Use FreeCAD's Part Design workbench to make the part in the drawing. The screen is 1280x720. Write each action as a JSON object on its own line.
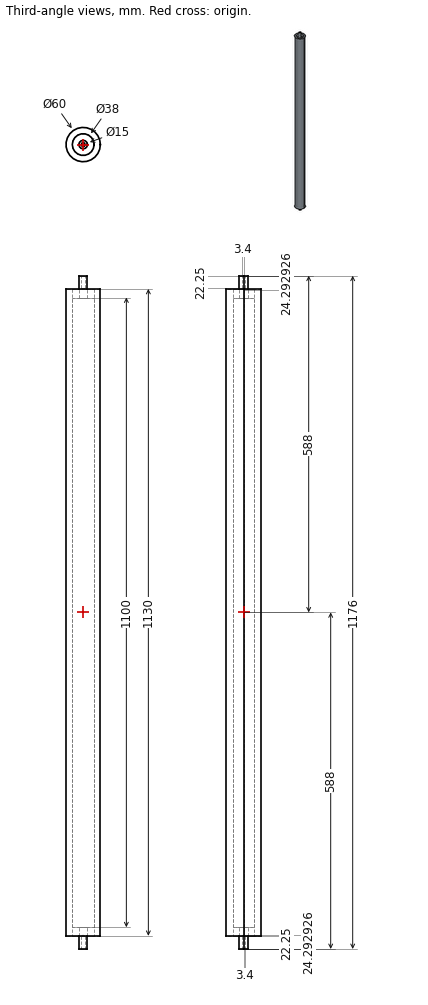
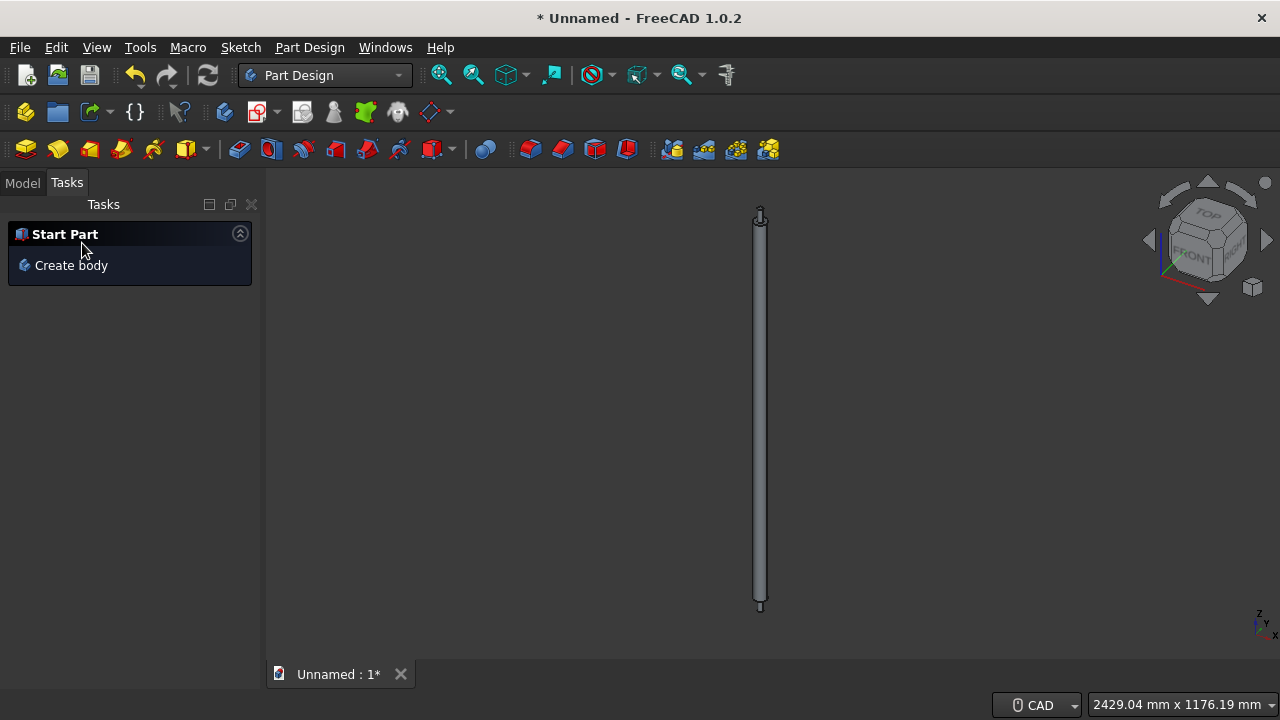
{"action": "left_click", "coordinate": [258, 112]}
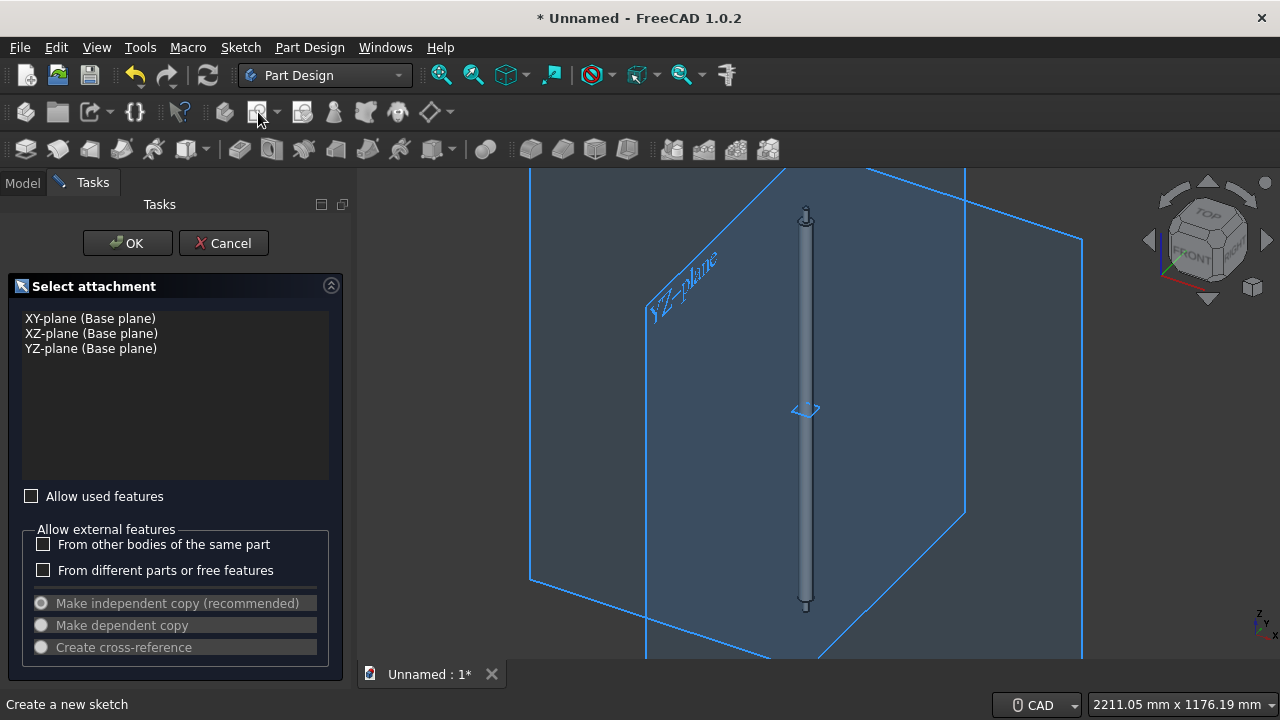
{"action": "left_click", "coordinate": [82, 348]}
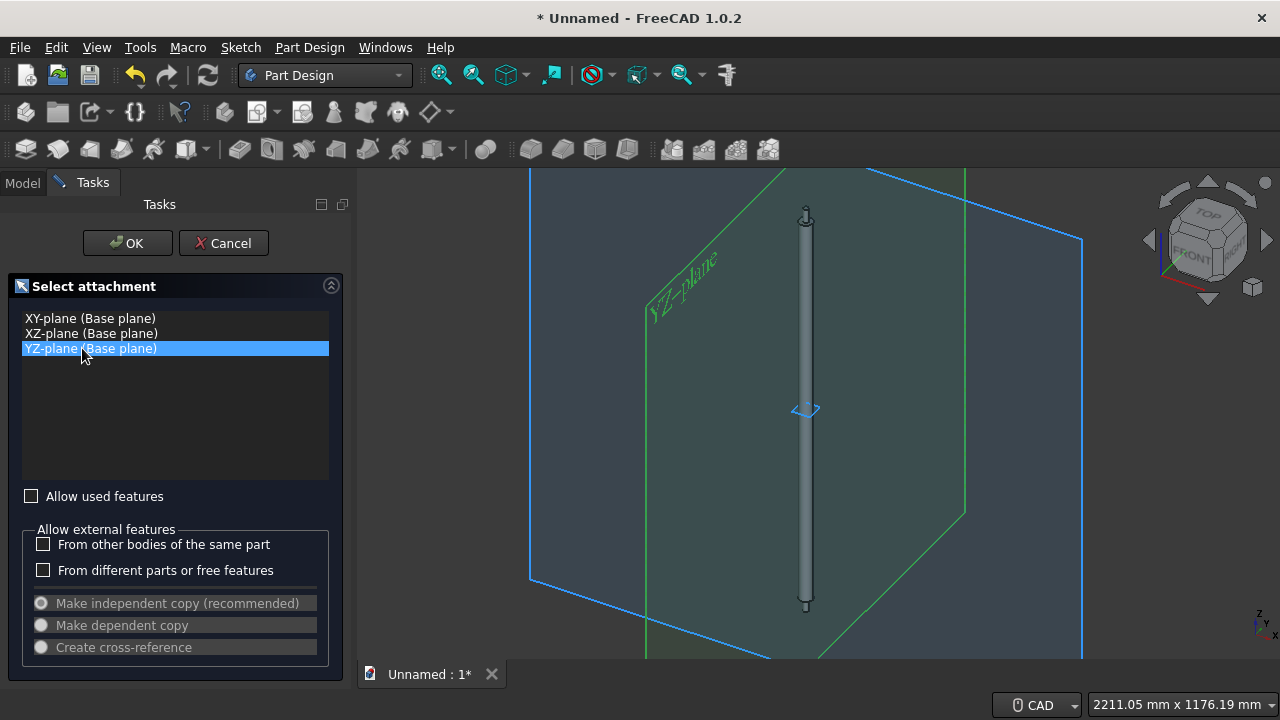
{"action": "left_click", "coordinate": [128, 243]}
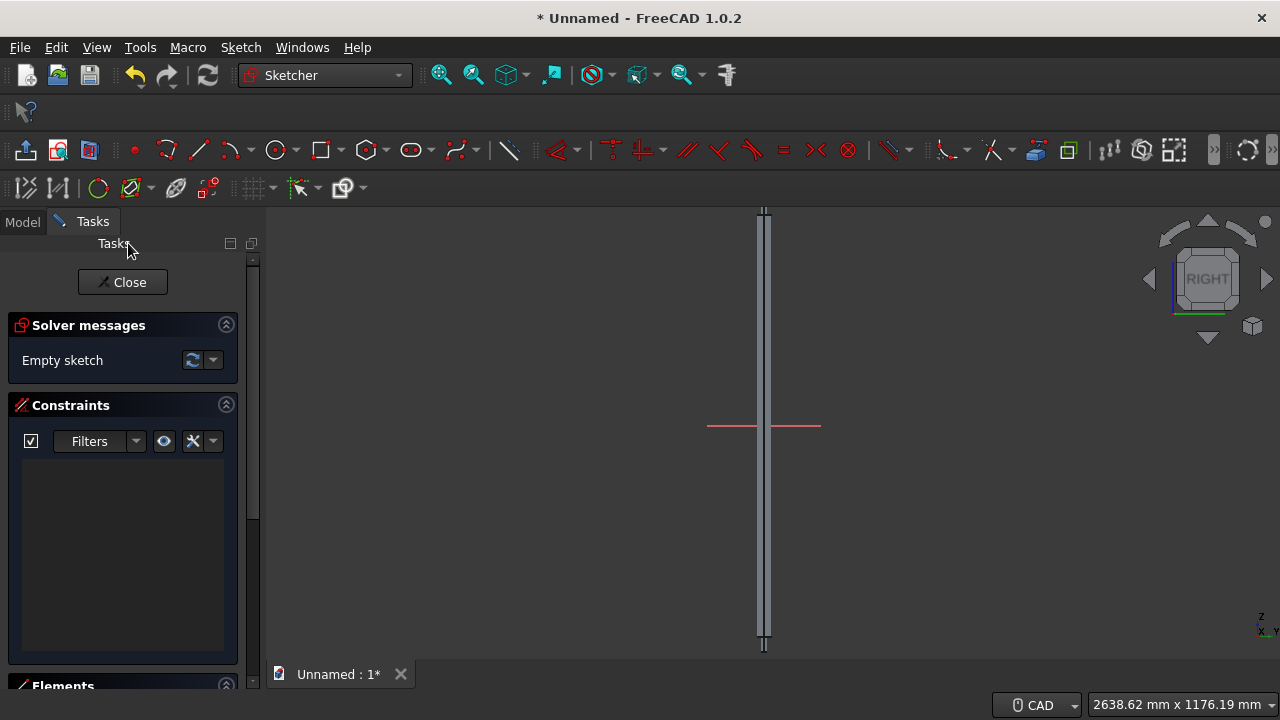
{"action": "key", "text": "q s"}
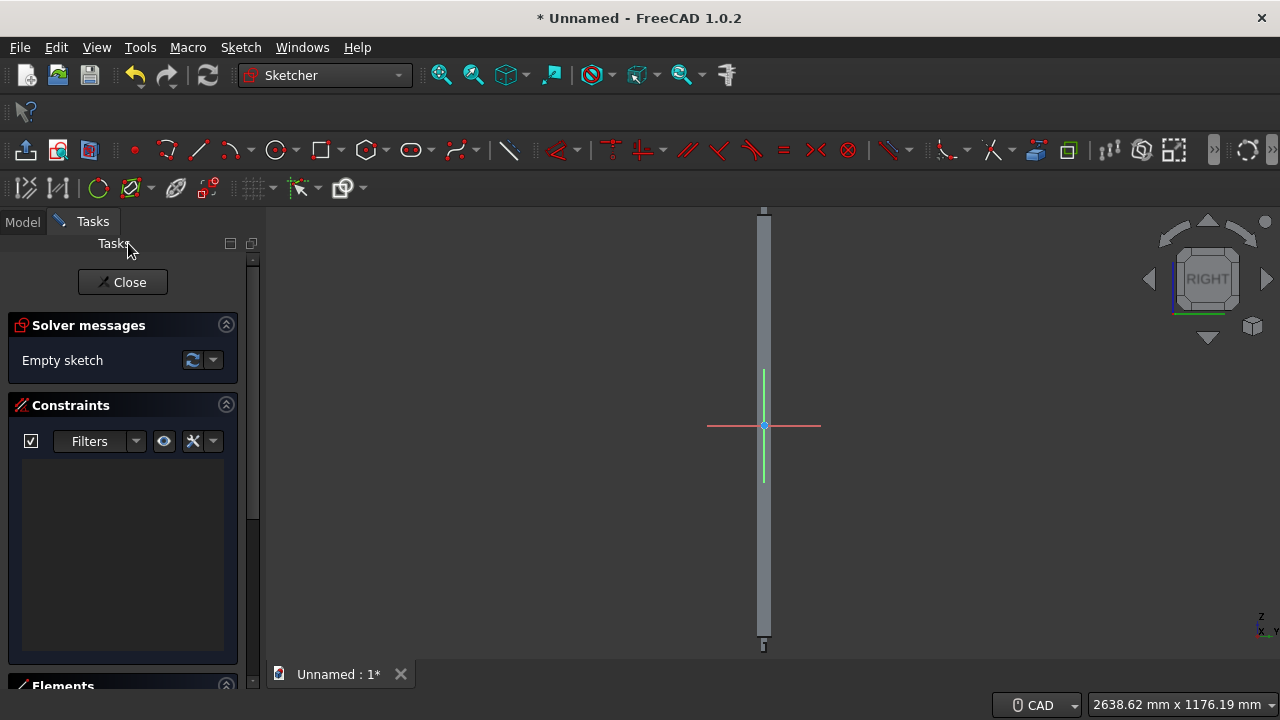
{"action": "scroll", "coordinate": [704, 433], "scroll_direction": "down", "scroll_amount": 5}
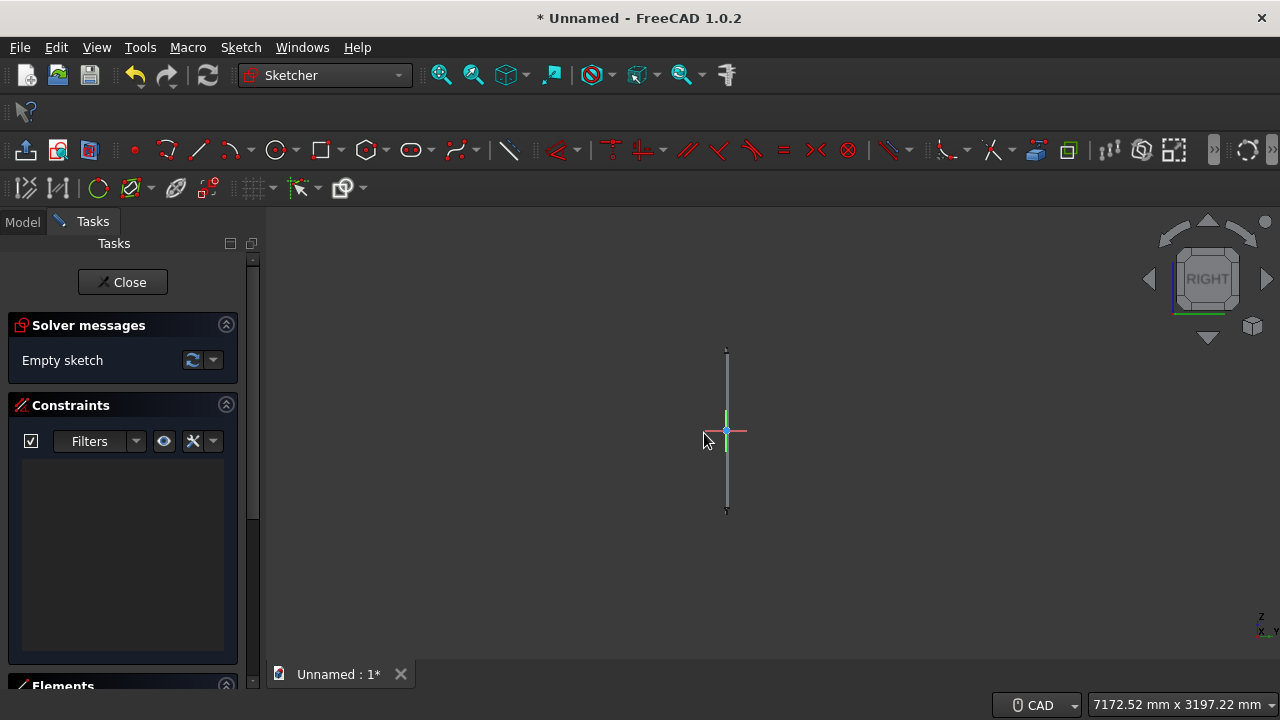
{"action": "scroll", "coordinate": [727, 345], "scroll_direction": "up", "scroll_amount": 15}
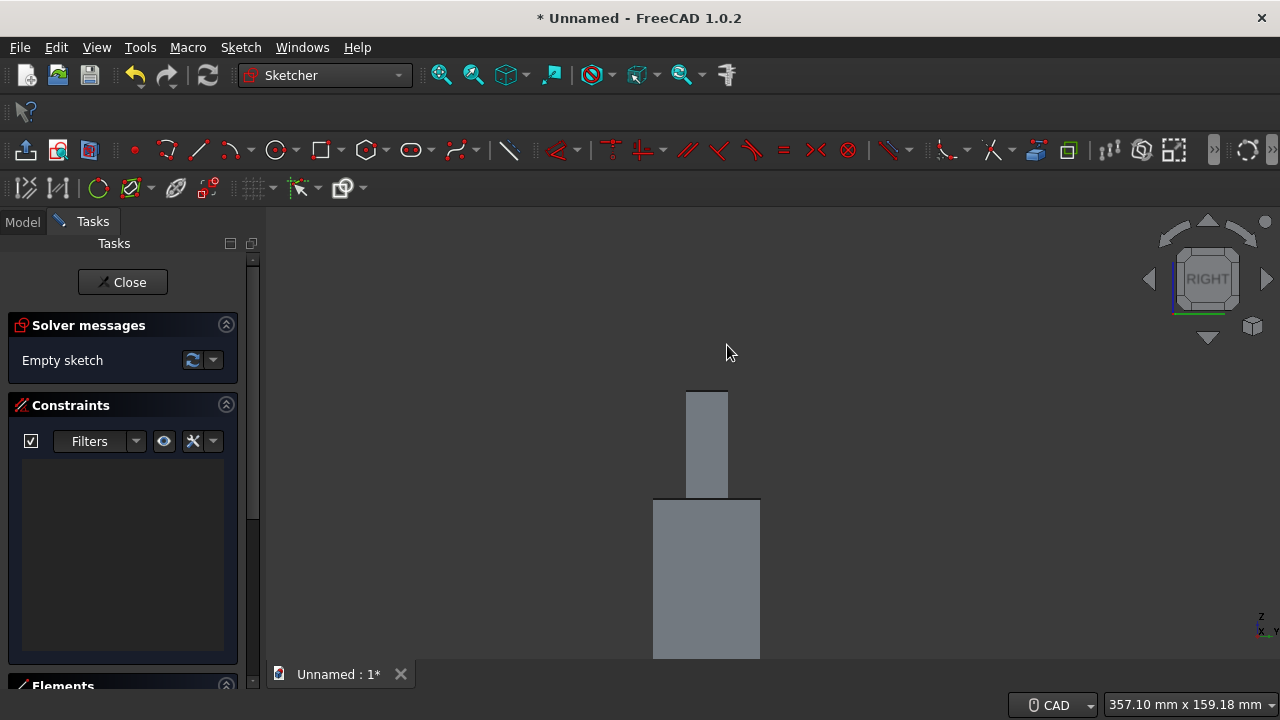
{"action": "scroll", "coordinate": [701, 423], "scroll_direction": "up", "scroll_amount": 7}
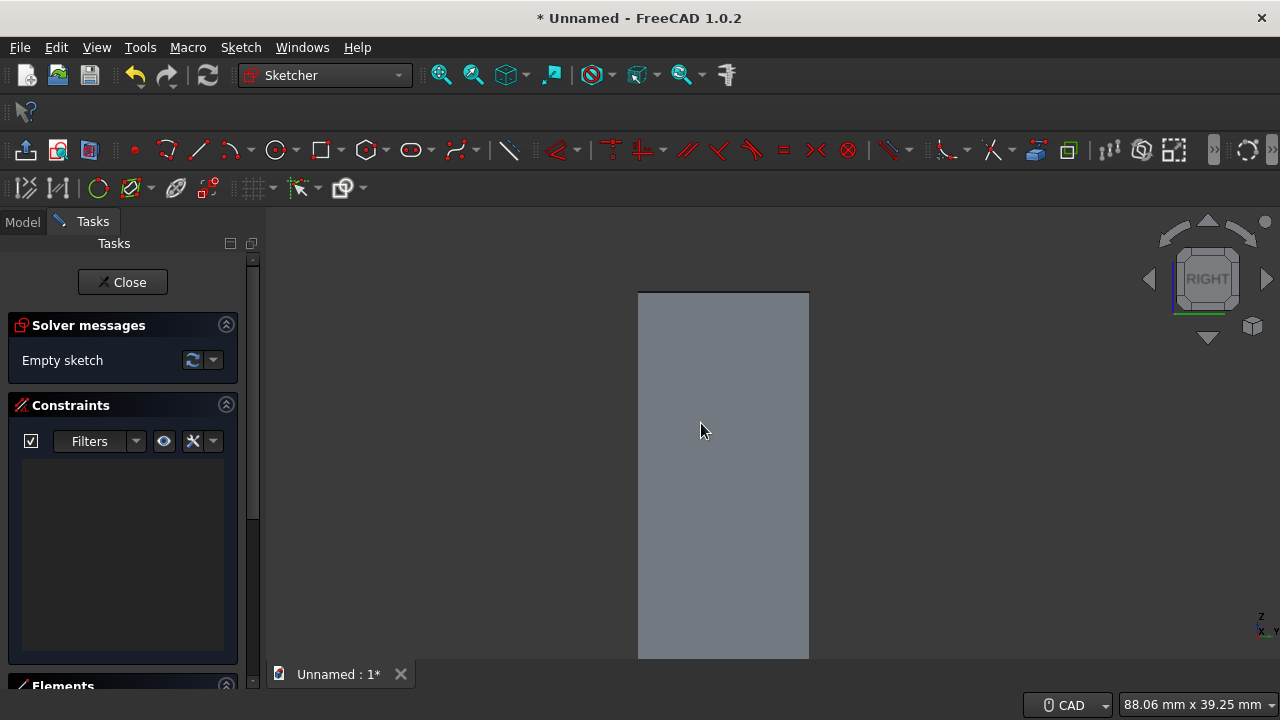
{"action": "key", "text": "g m"}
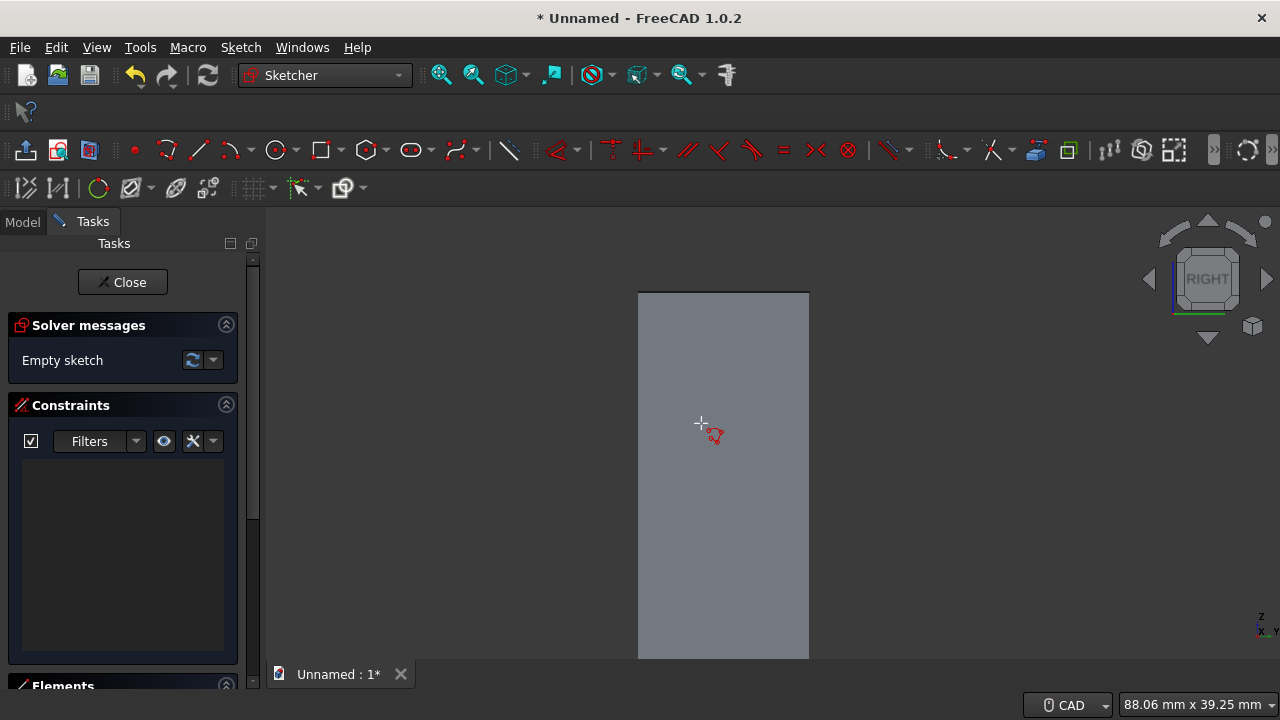
{"action": "left_click", "coordinate": [724, 572]}
{"action": "left_click", "coordinate": [715, 292]}
{"action": "left_click", "coordinate": [685, 292]}
{"action": "left_click", "coordinate": [685, 548]}
{"action": "left_click", "coordinate": [724, 573]}
{"action": "key", "text": "Escape"}
{"action": "key", "text": "Escape"}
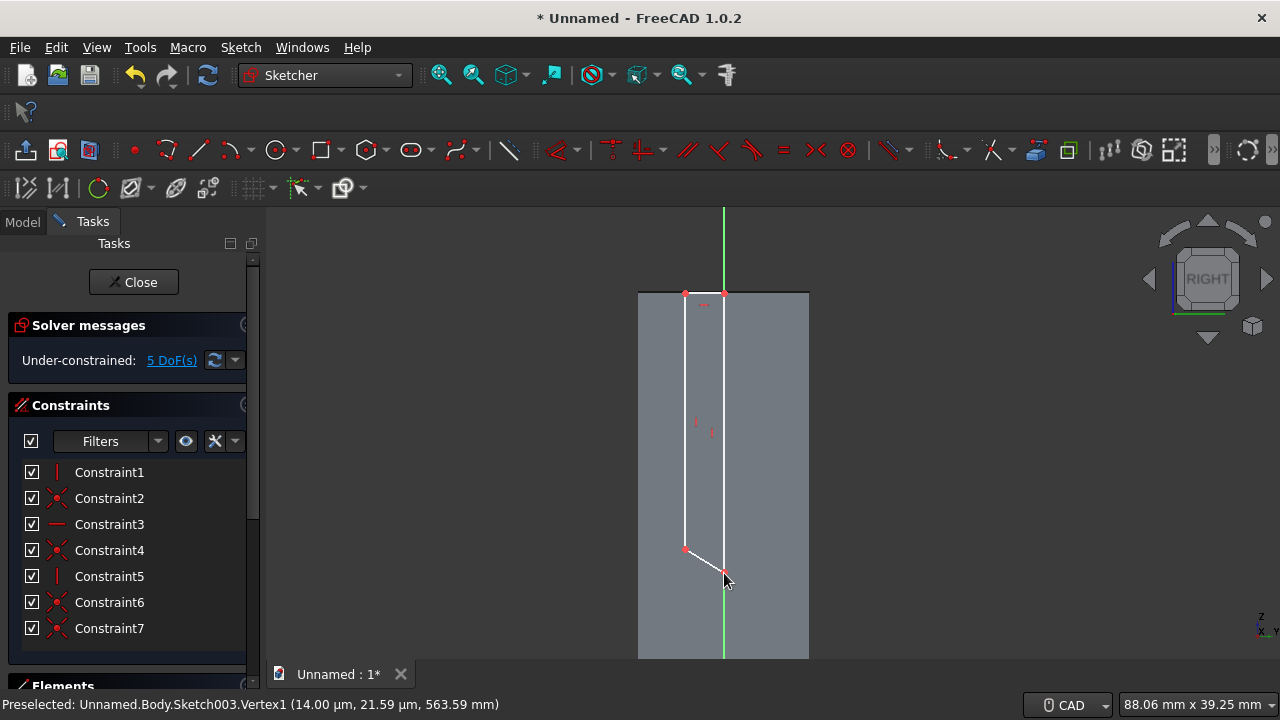
{"action": "left_click", "coordinate": [724, 573]}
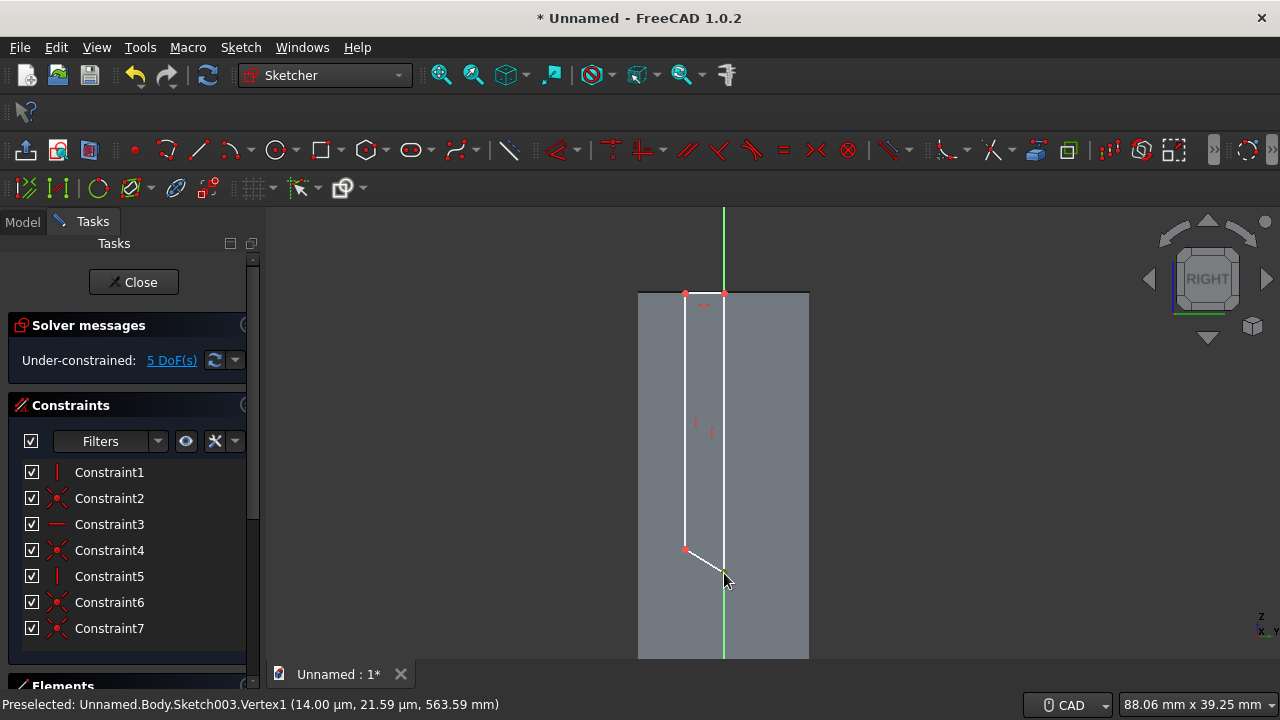
{"action": "left_click", "coordinate": [724, 603]}